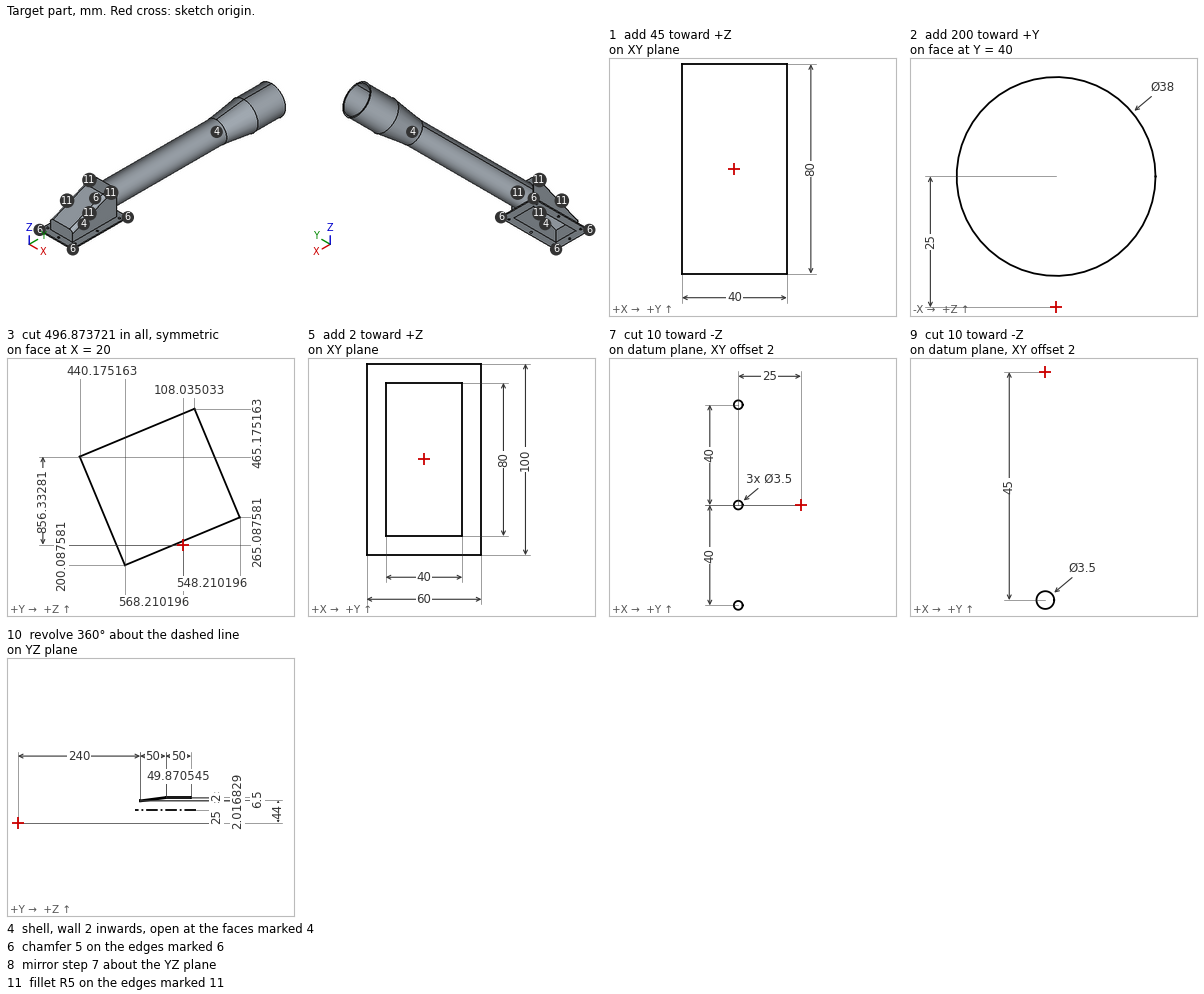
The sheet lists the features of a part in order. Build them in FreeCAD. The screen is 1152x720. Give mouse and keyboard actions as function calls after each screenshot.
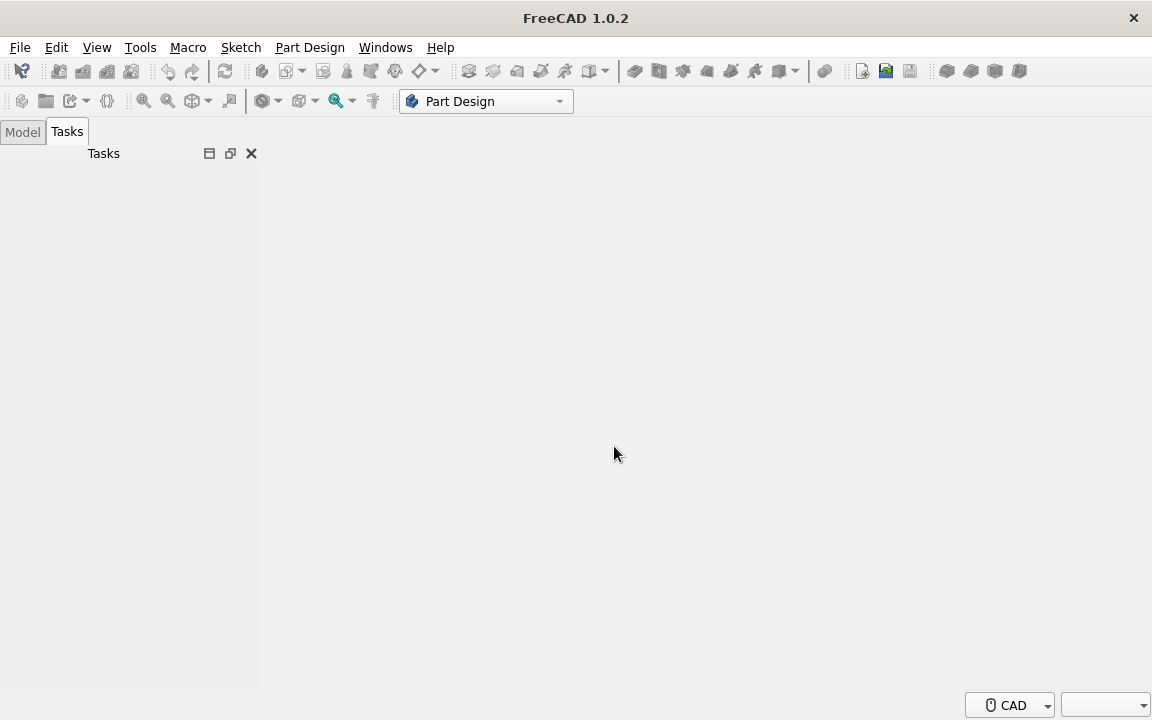
key(ctrl+n)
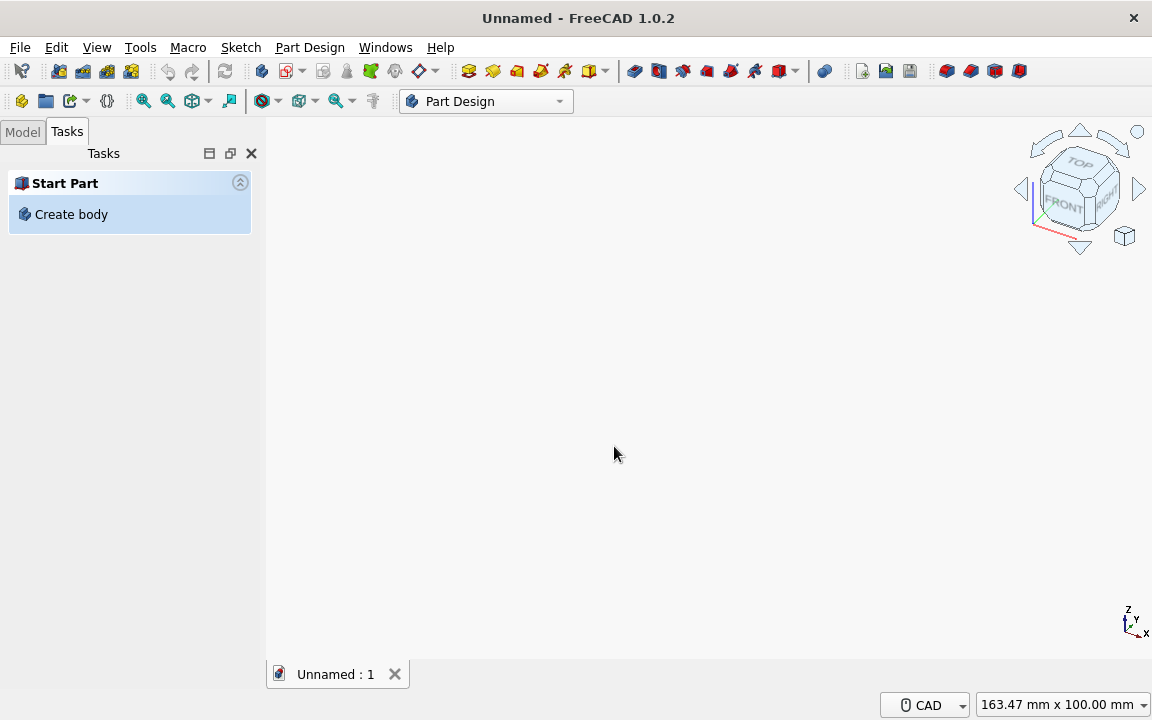
click(286, 72)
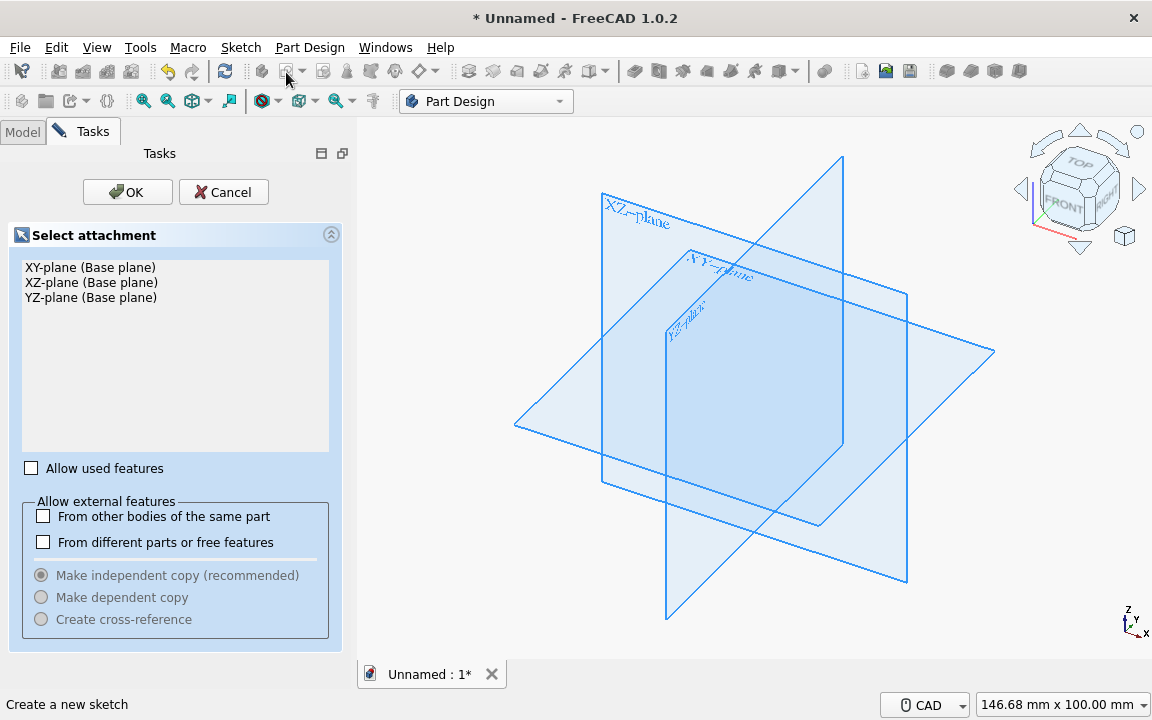
click(82, 268)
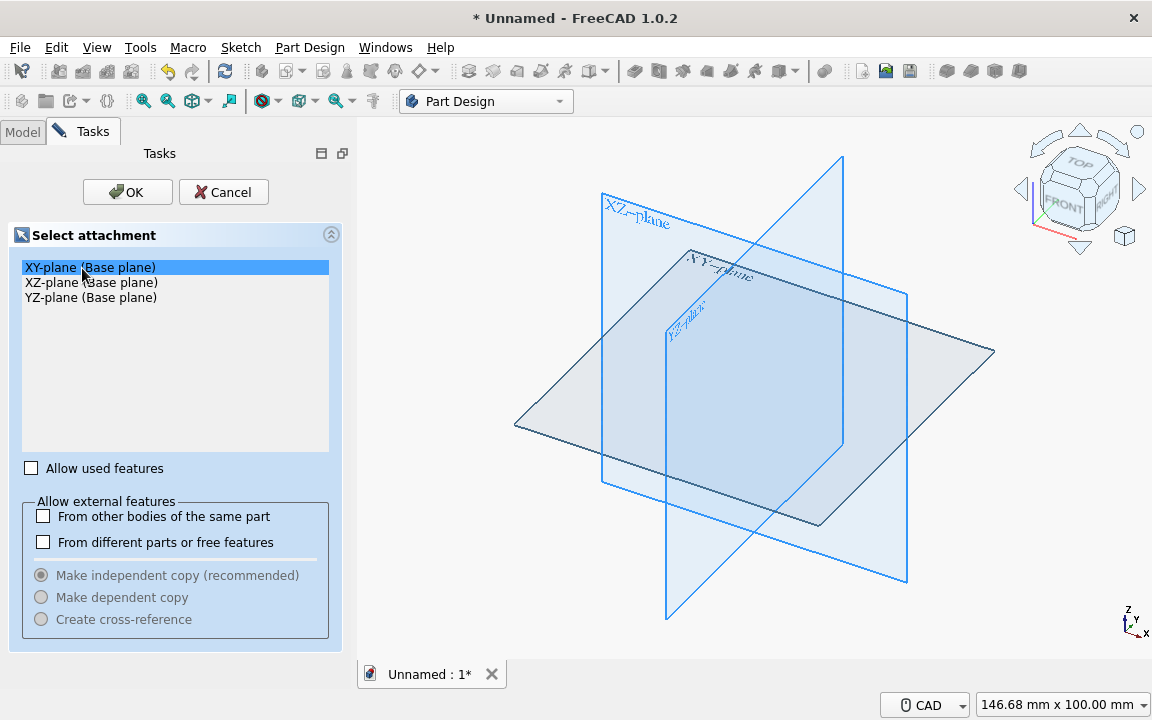
click(128, 192)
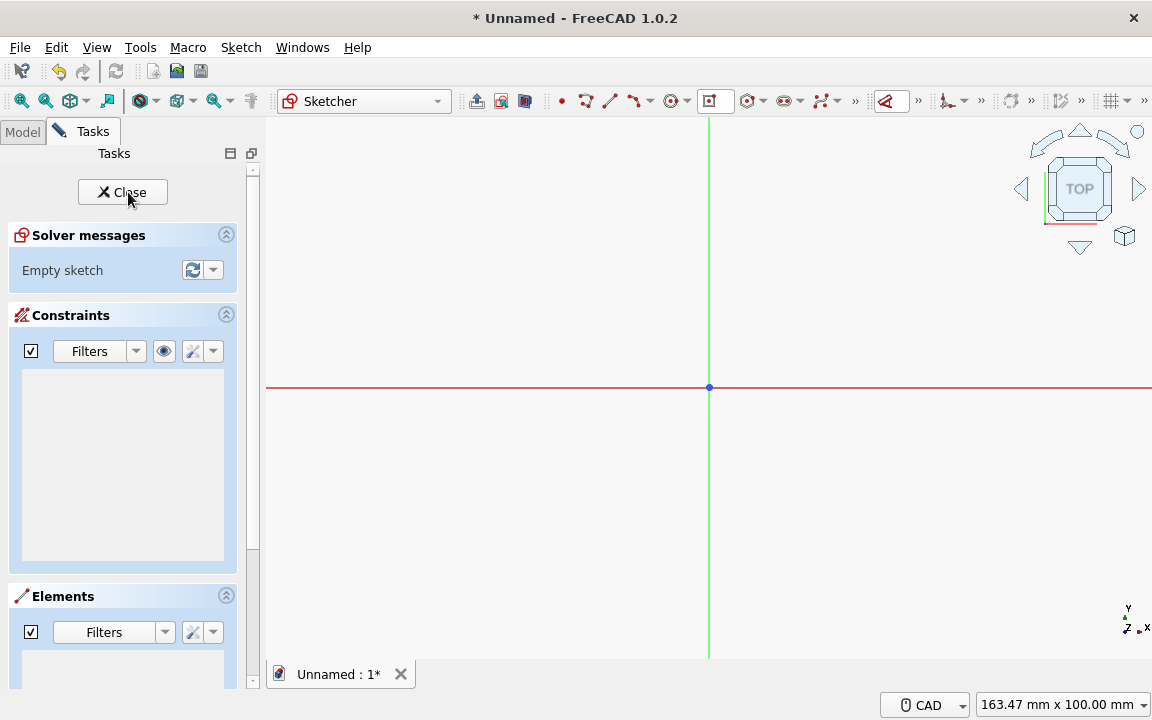
key(g)
key(v)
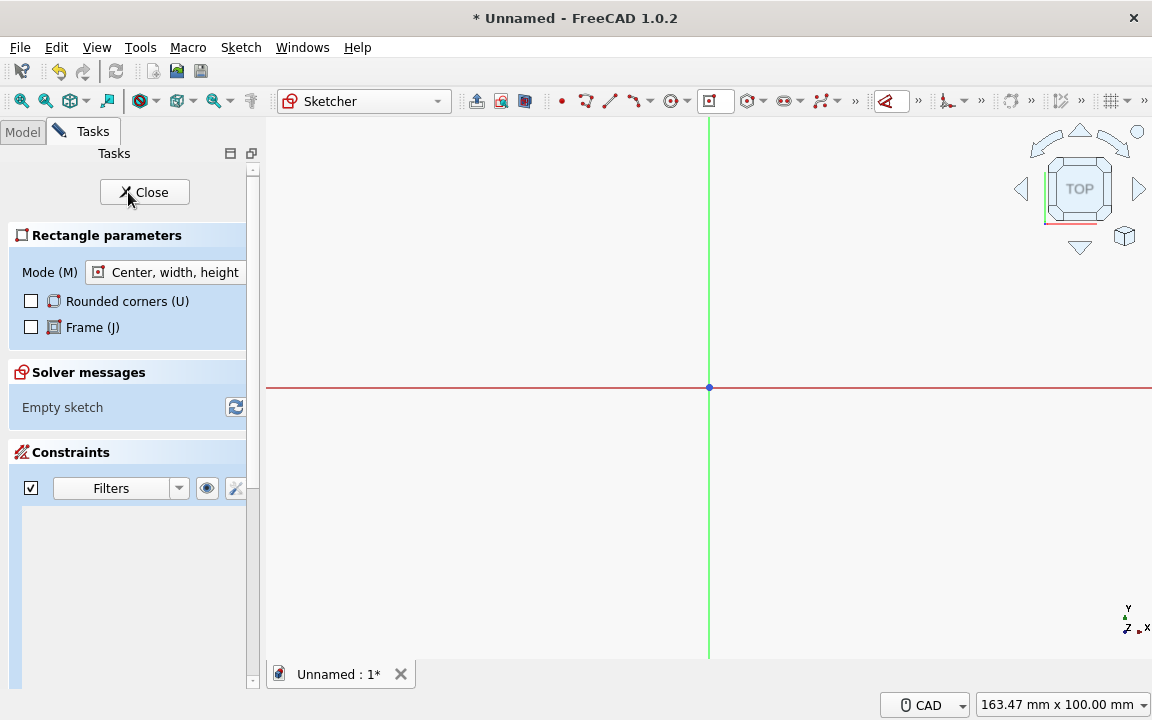
click(709, 388)
move(817, 171)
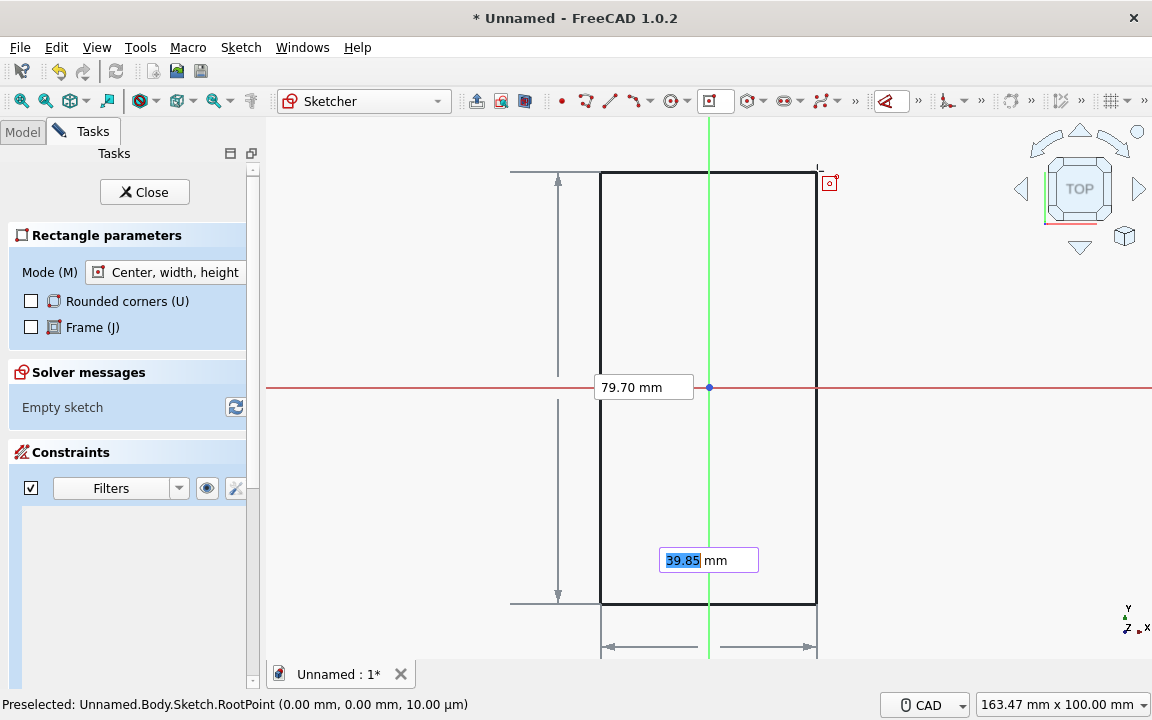
text(40)
key(Tab)
text(80)
key(Return)
key(Escape)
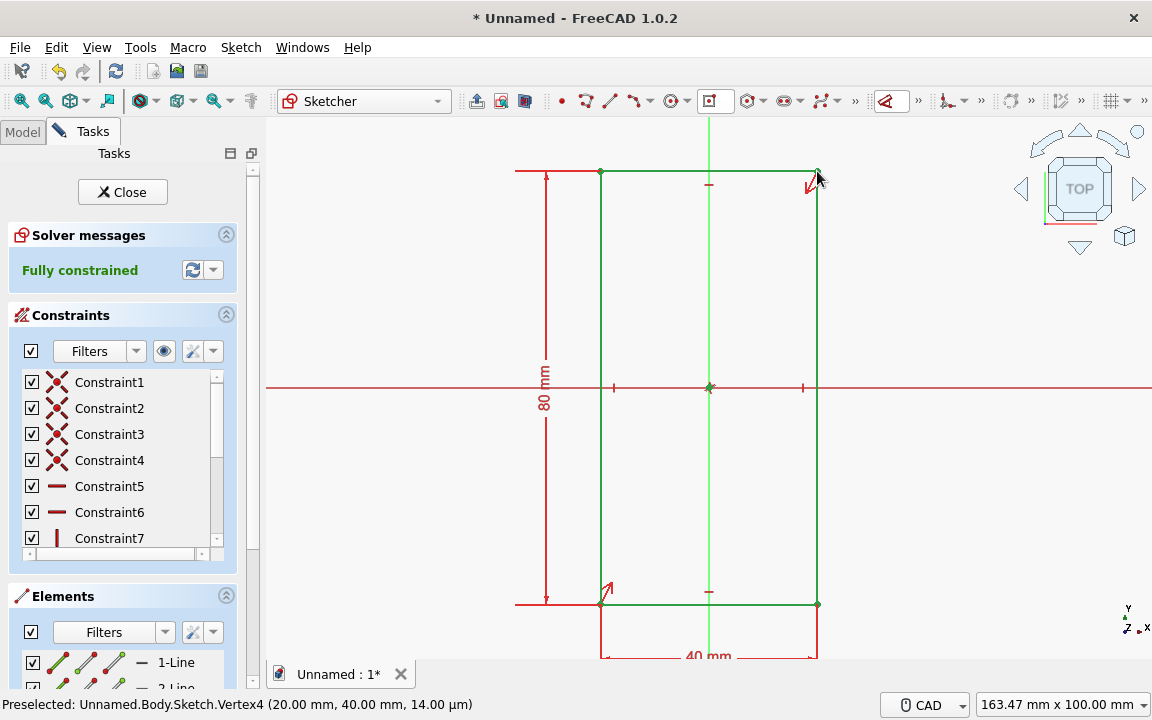
click(123, 192)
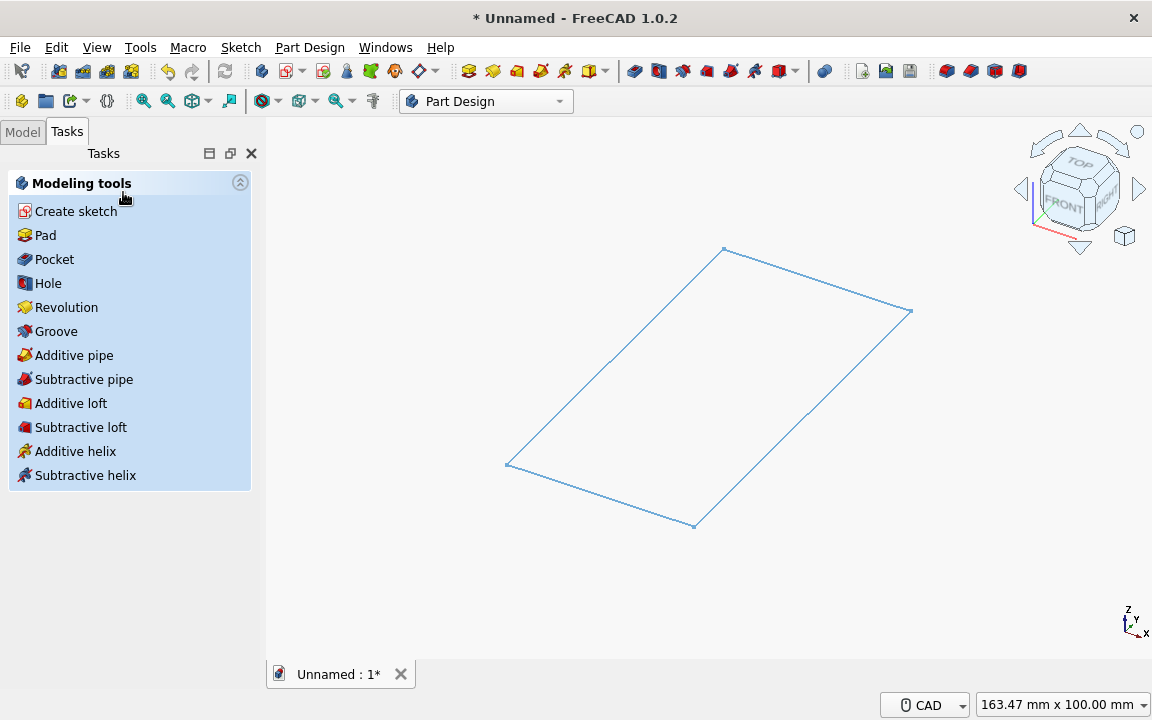
click(470, 72)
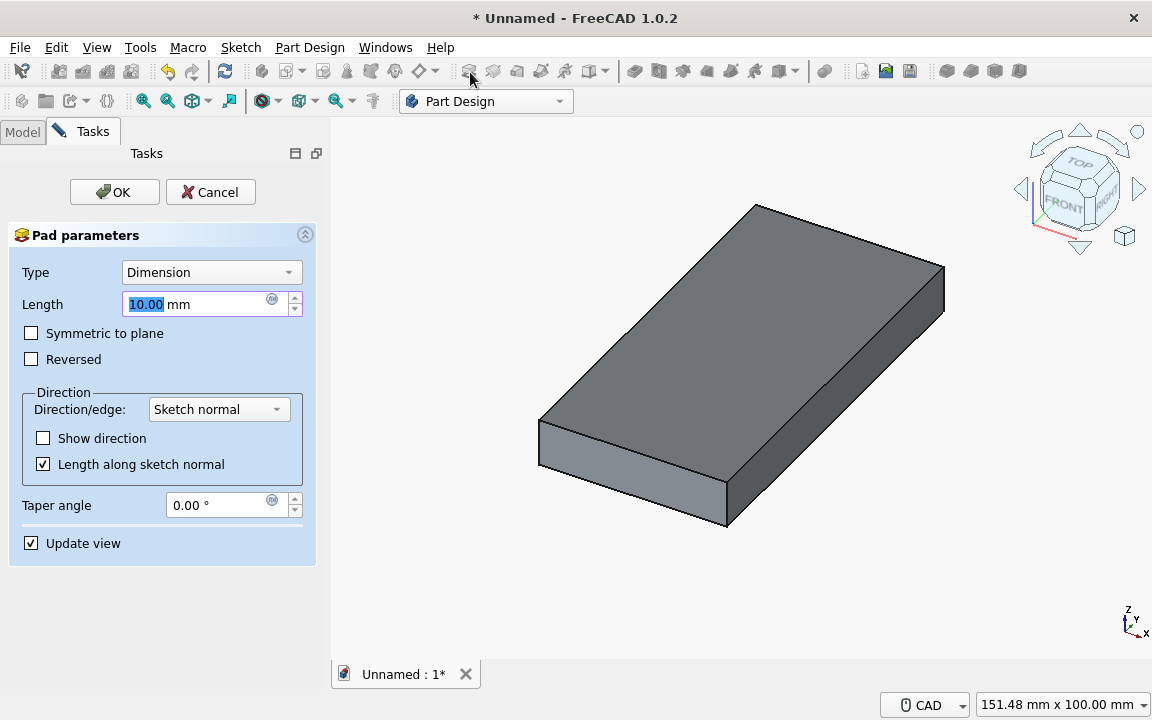
text(45)
key(Tab)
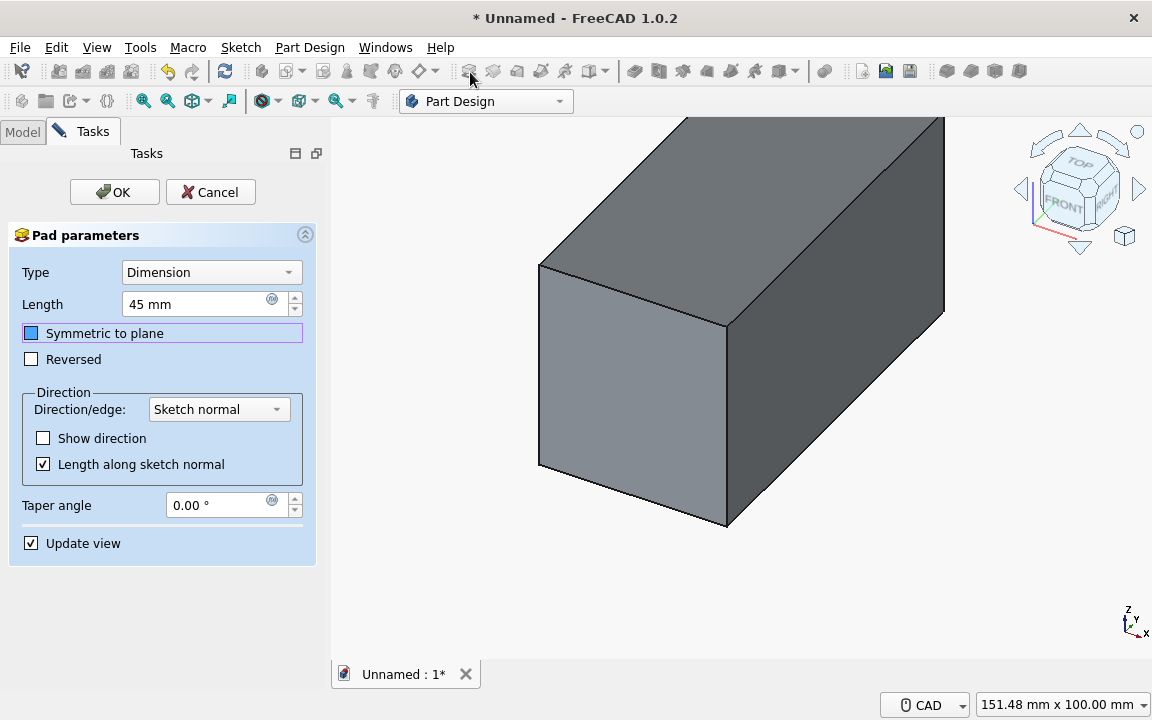
click(115, 192)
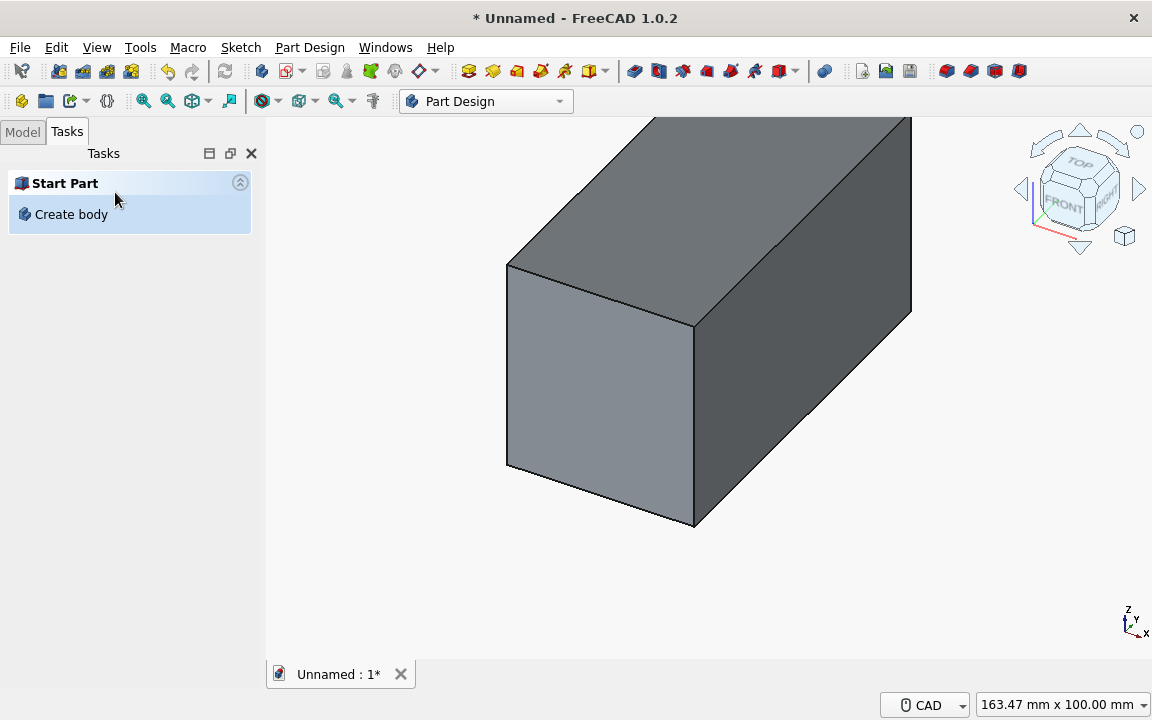
key(v)
key(f)